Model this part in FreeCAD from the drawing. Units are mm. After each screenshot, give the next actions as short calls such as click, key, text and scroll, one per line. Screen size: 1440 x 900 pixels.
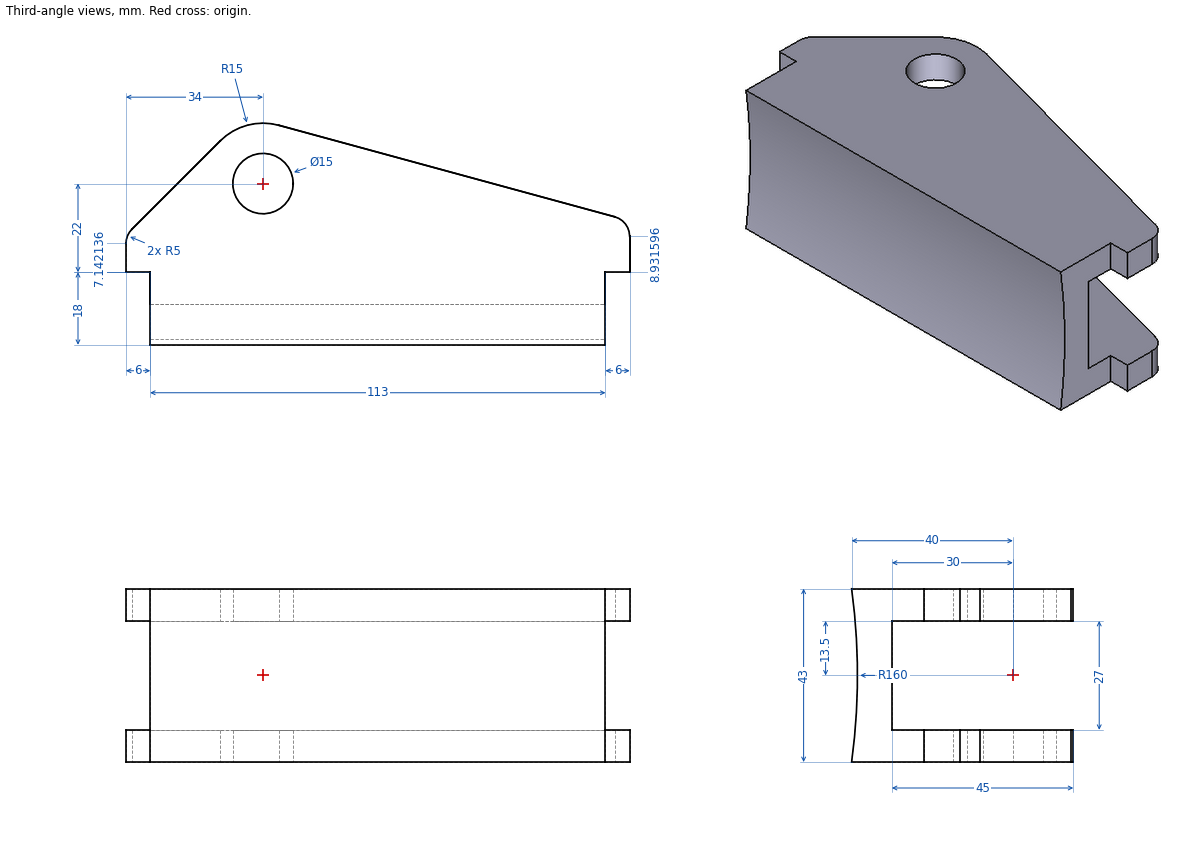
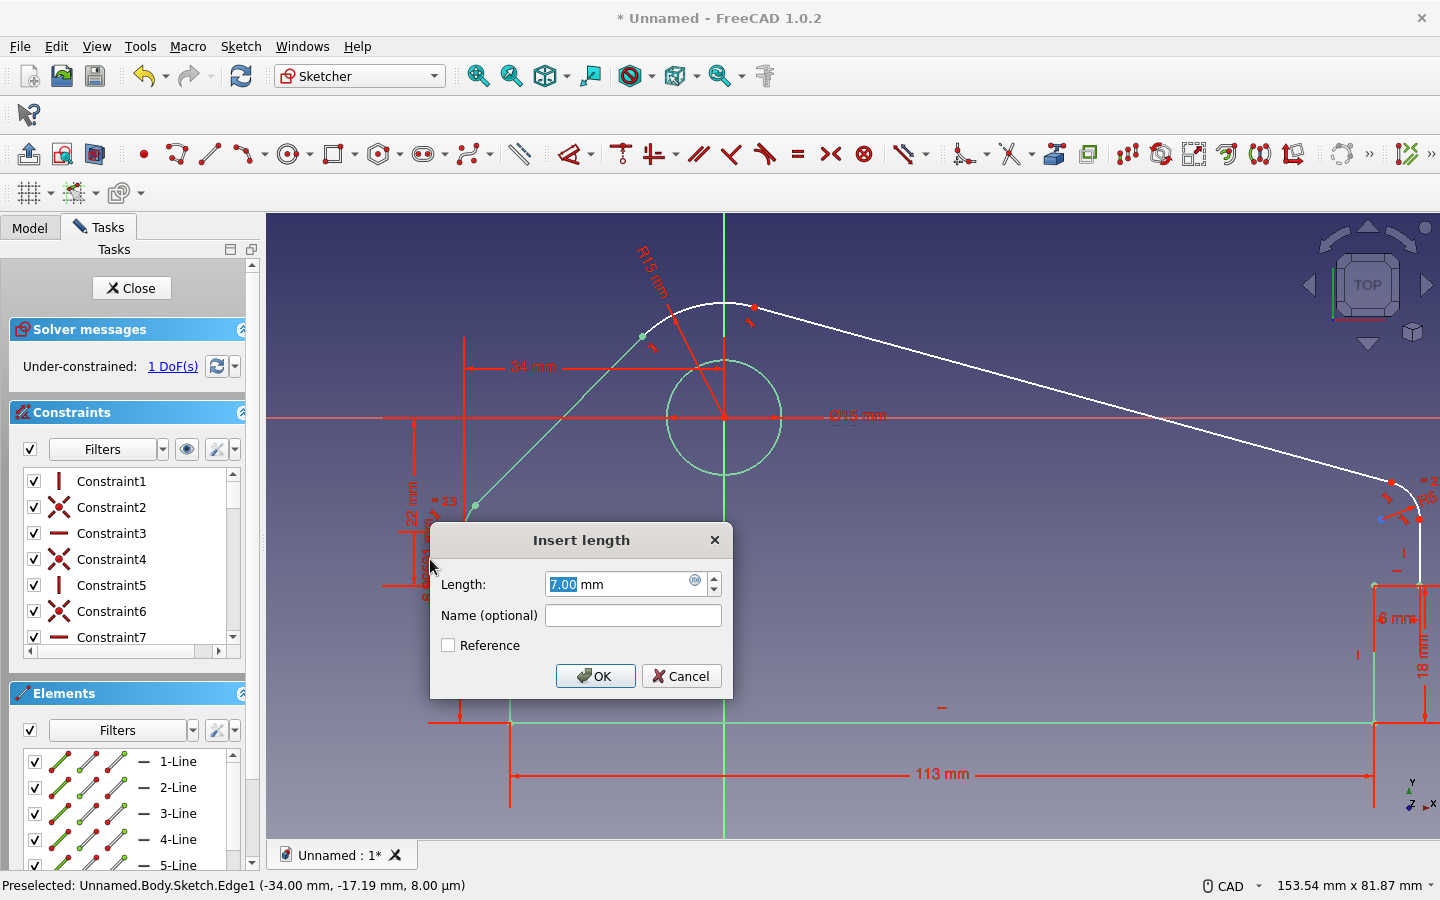
text(7.142136)
key(Return)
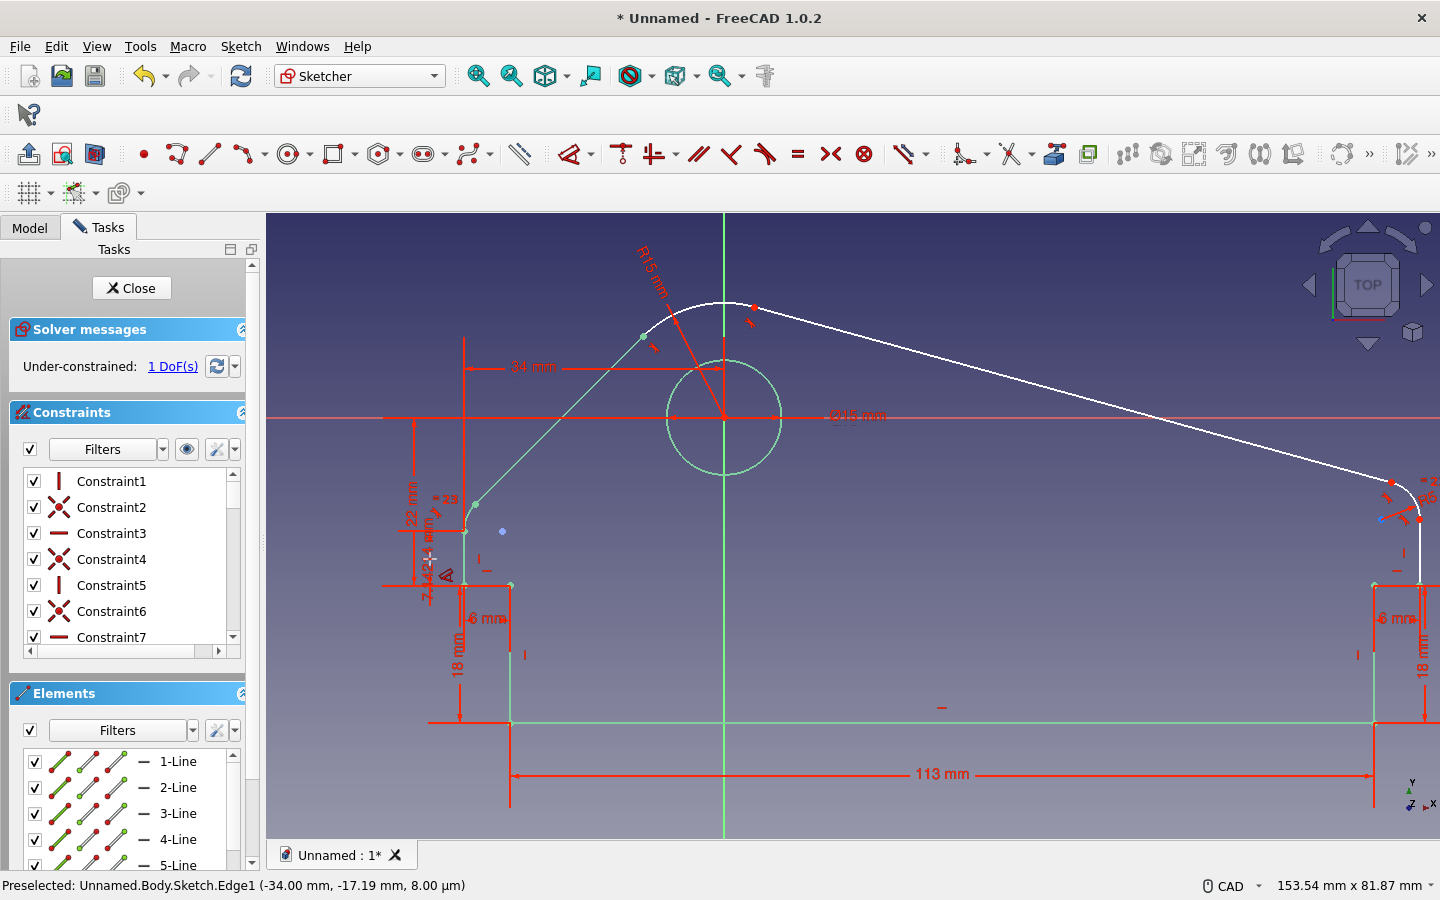
scroll(464, 548, down, 2)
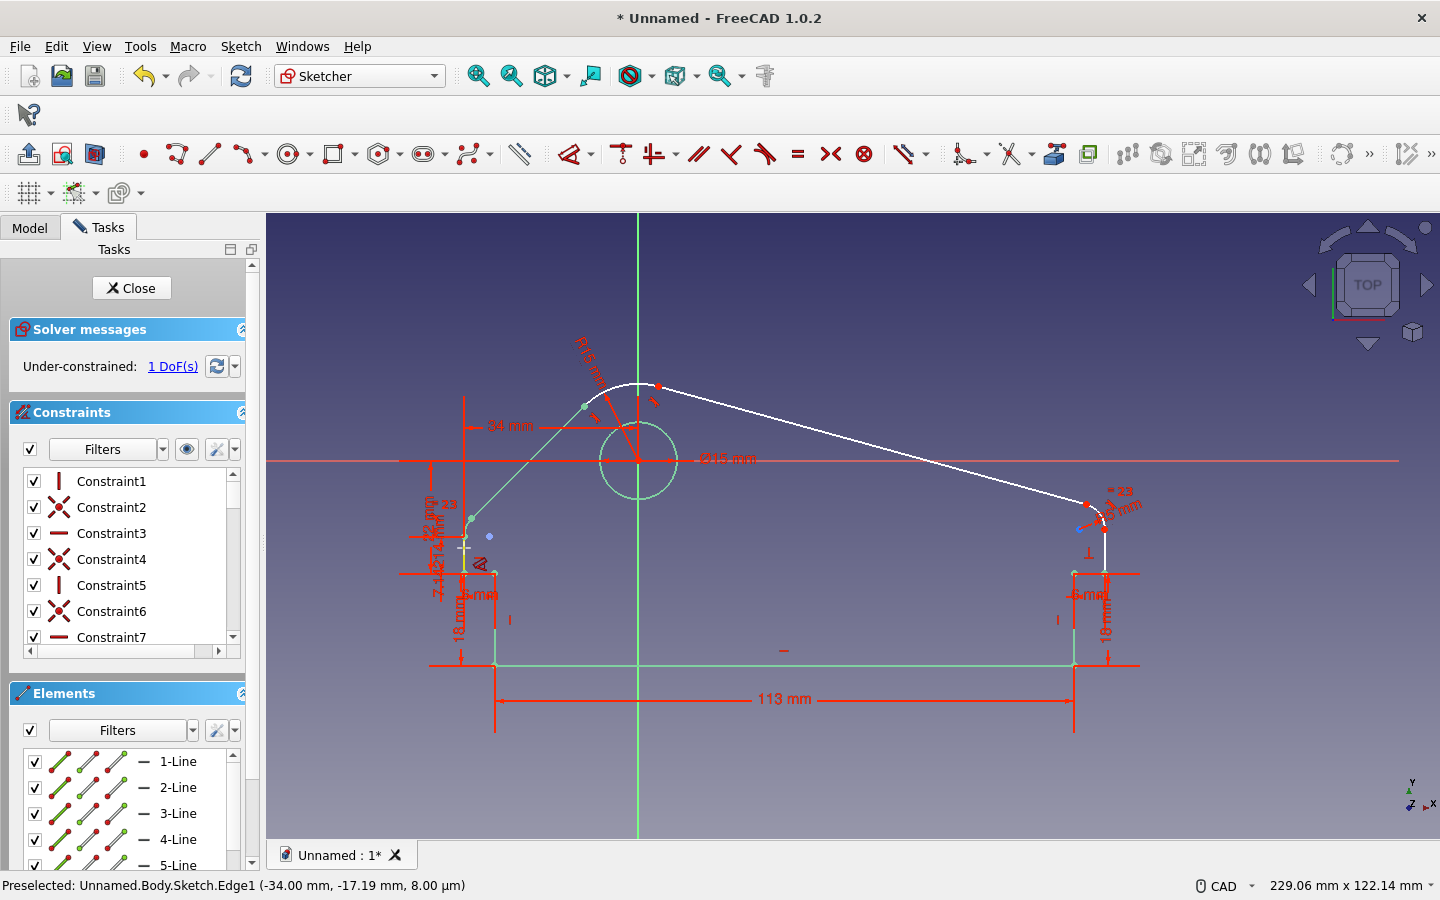
click(1105, 560)
click(1139, 551)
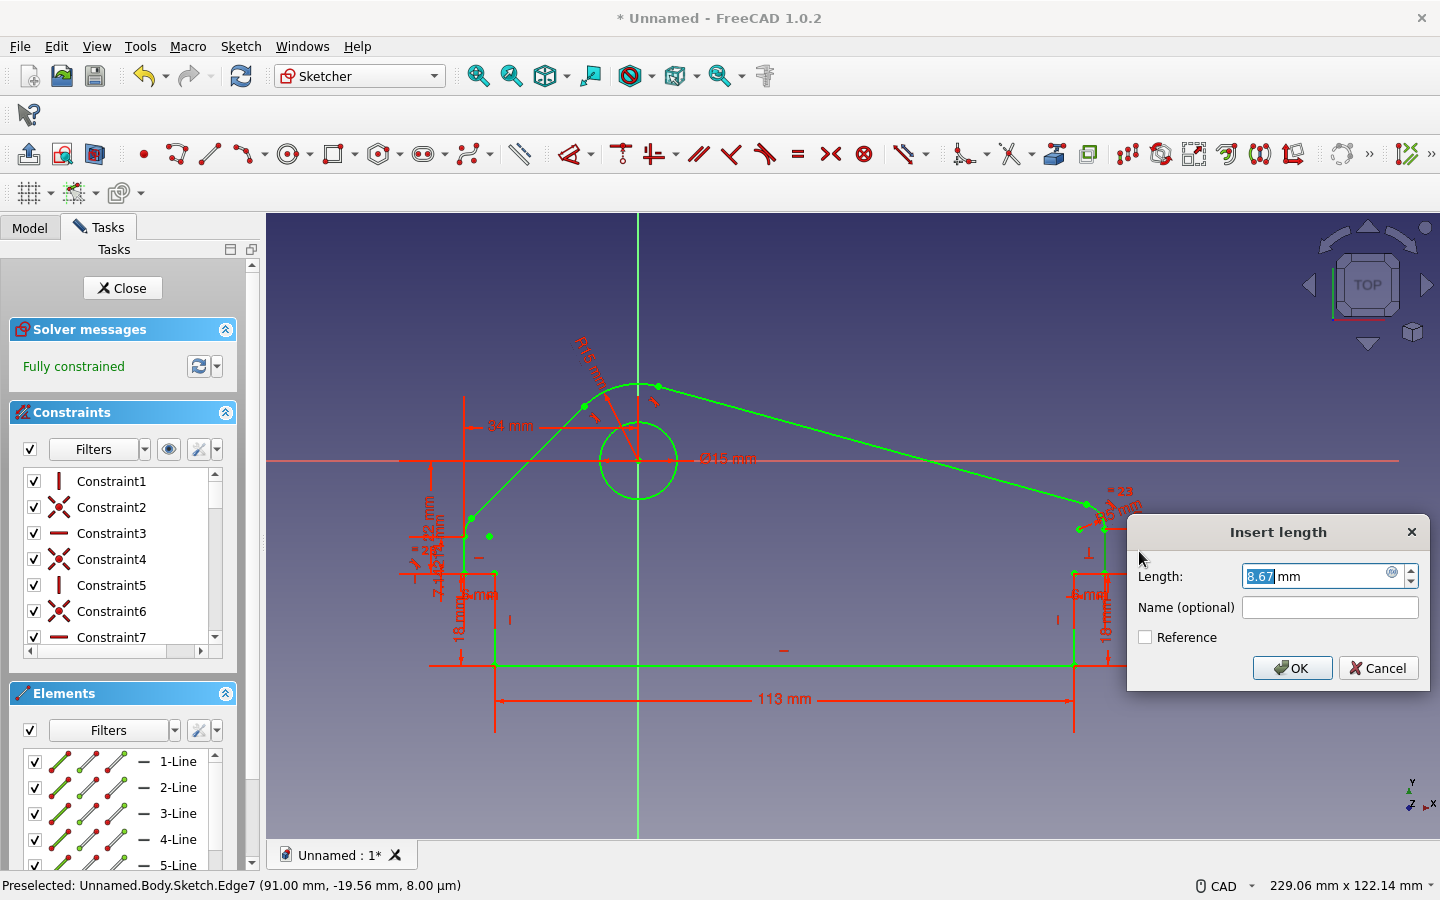
text(8.931596)
key(Return)
key(Escape)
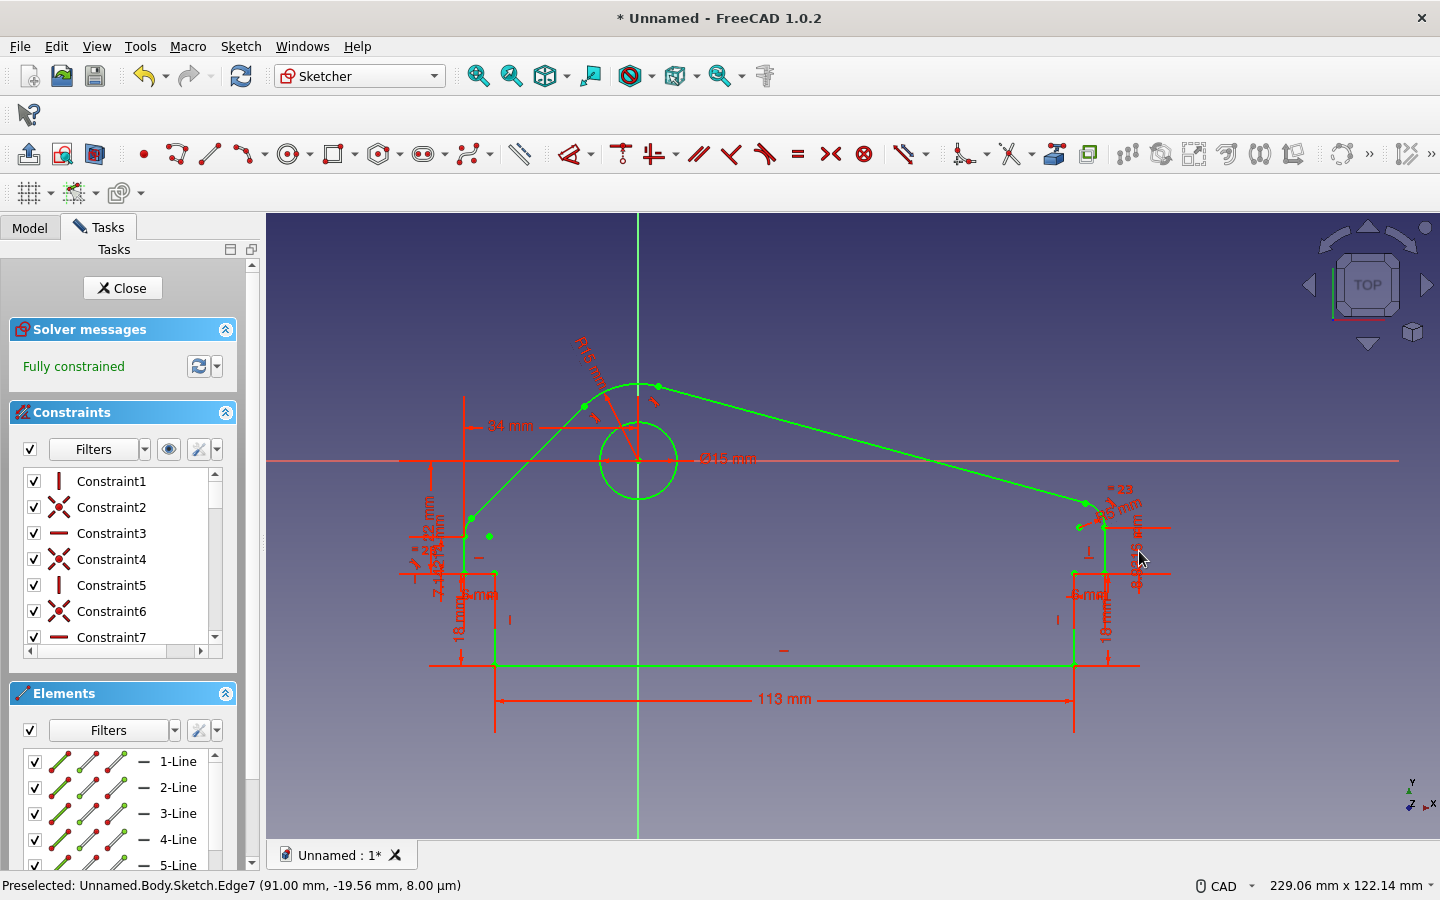
click(123, 288)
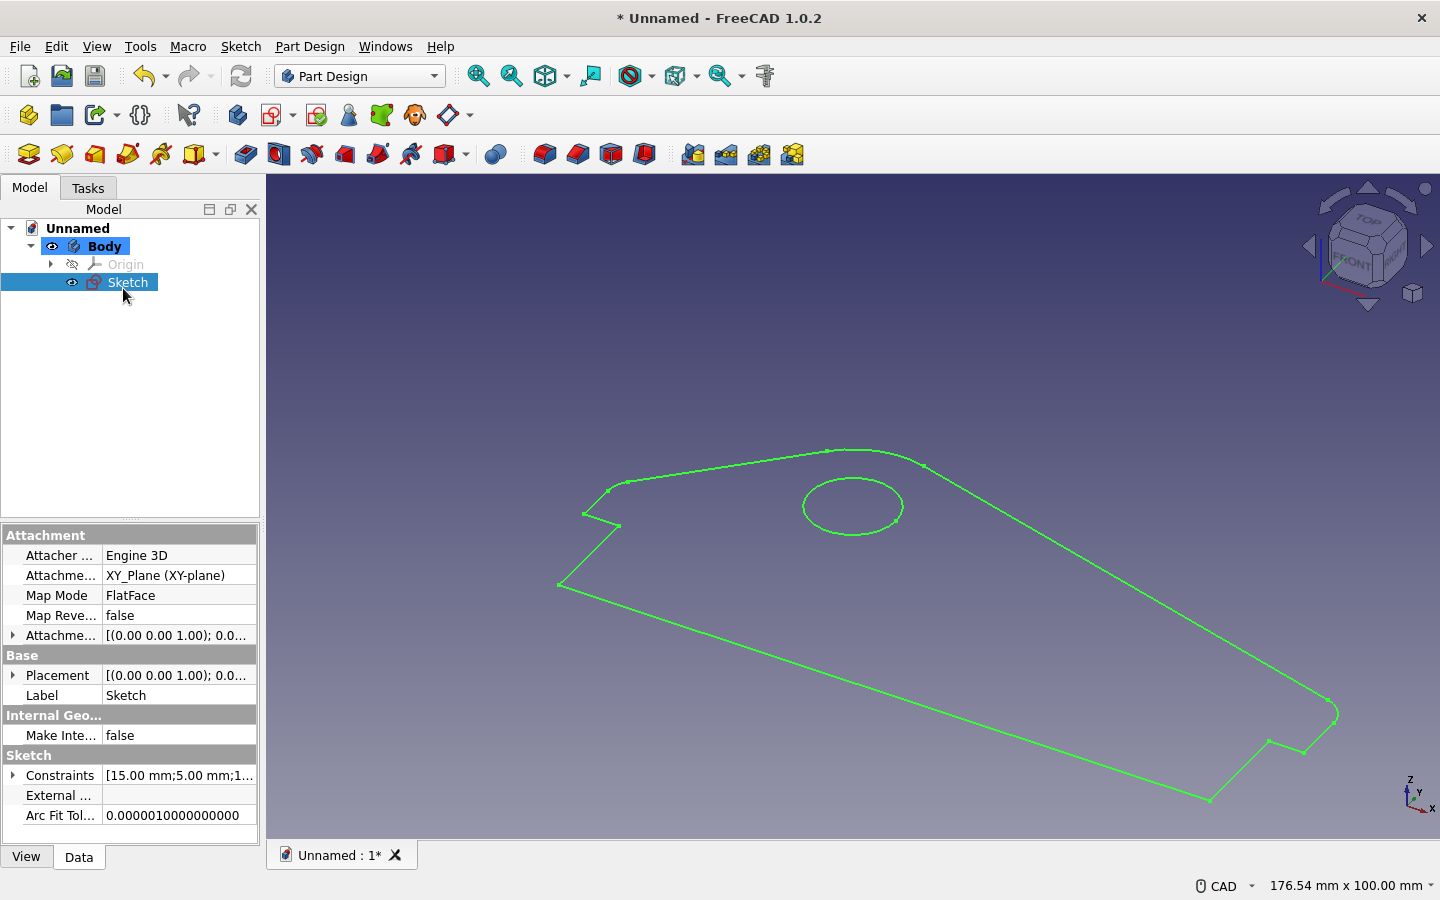
click(29, 154)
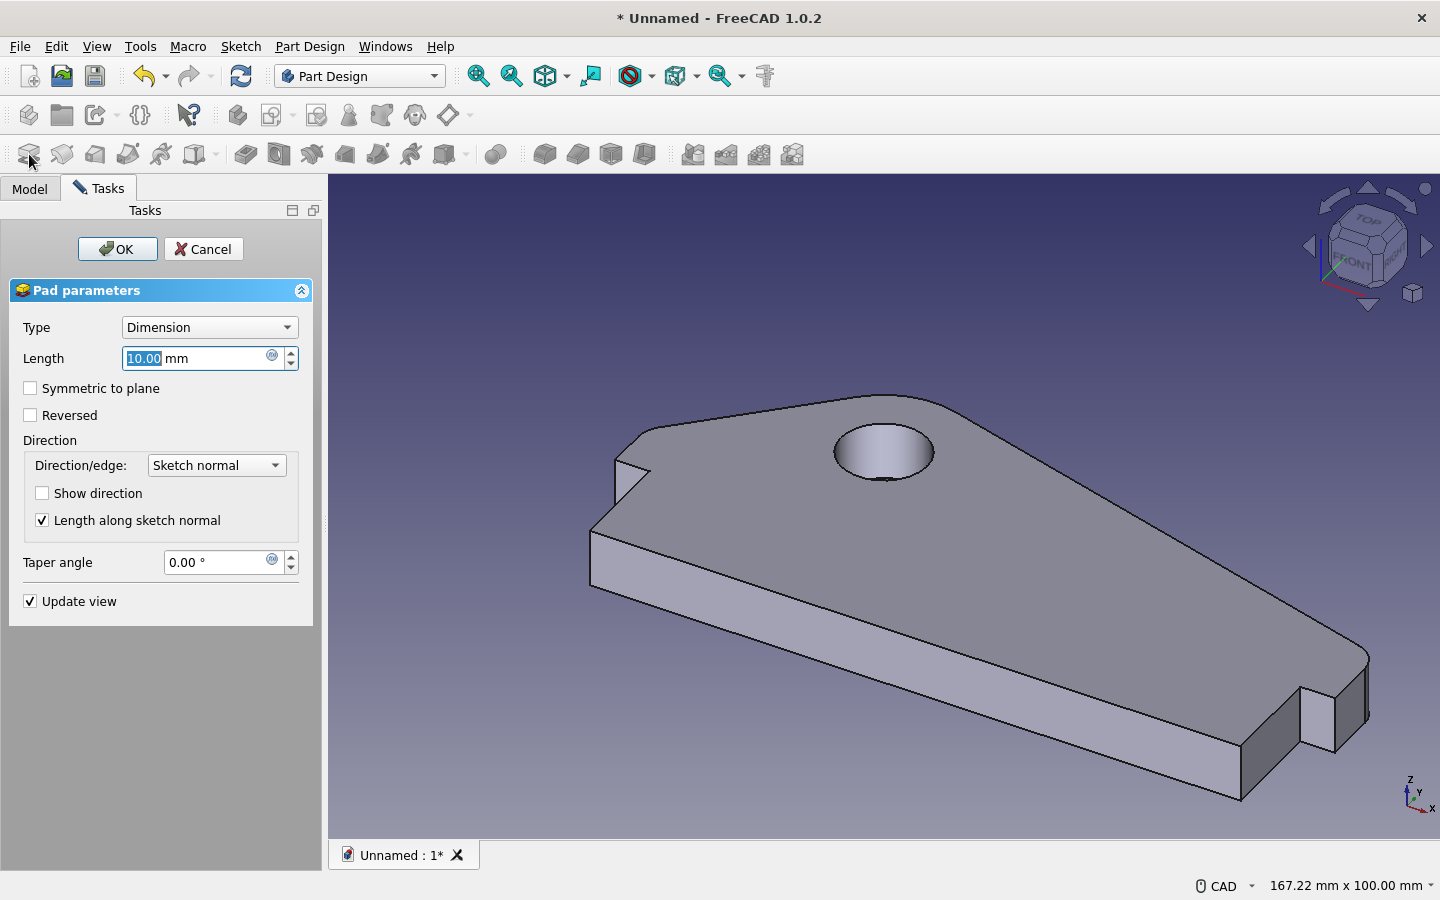
text(43)
key(Tab)